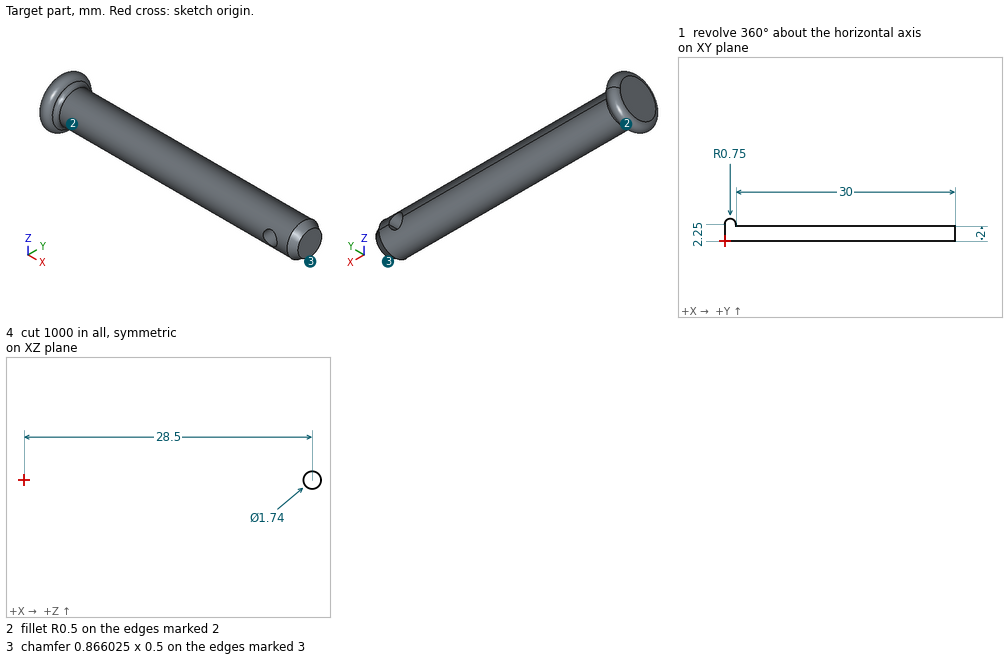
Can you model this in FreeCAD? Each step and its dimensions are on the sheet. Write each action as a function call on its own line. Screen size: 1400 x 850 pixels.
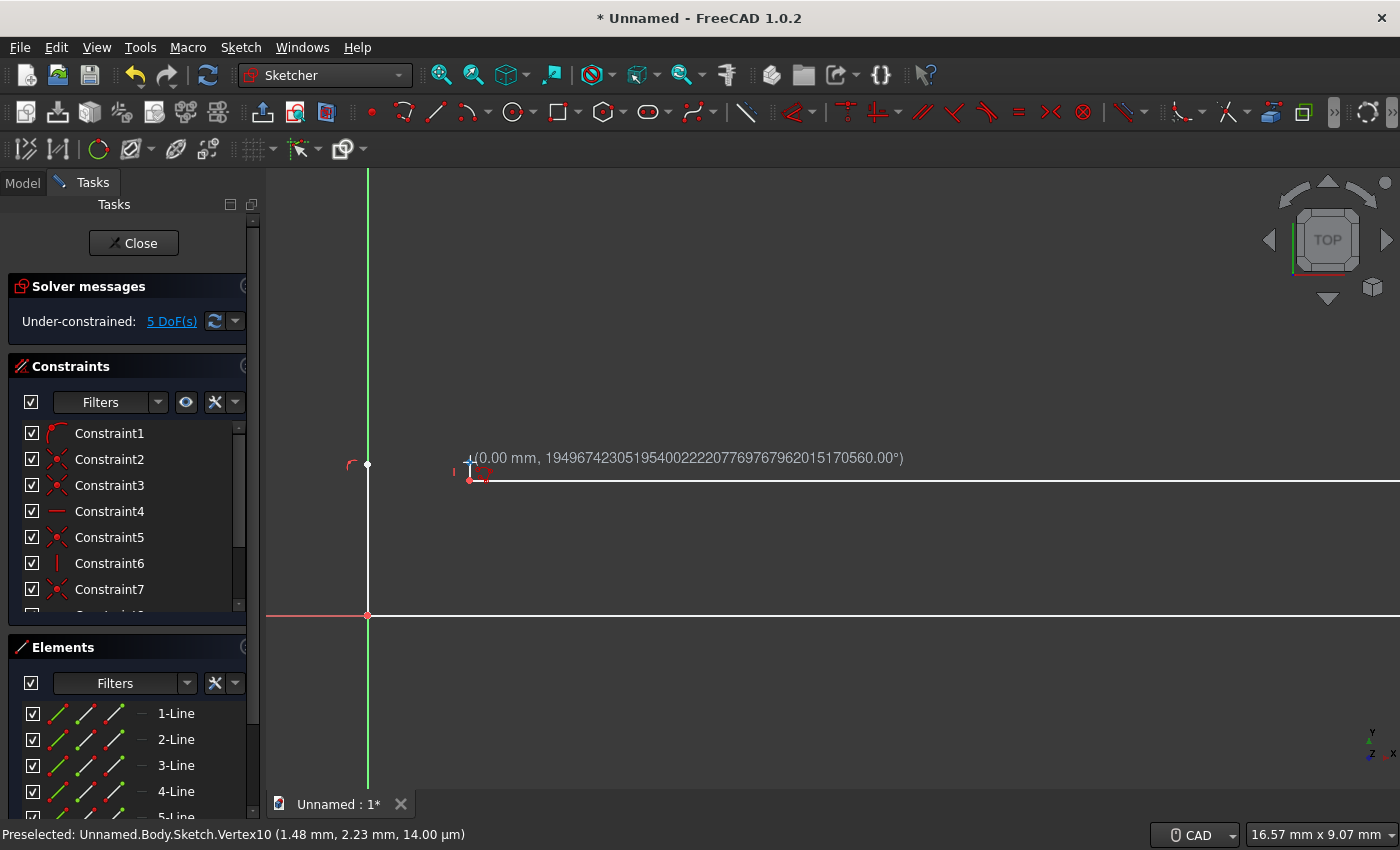
key(g)
key(3)
key(a)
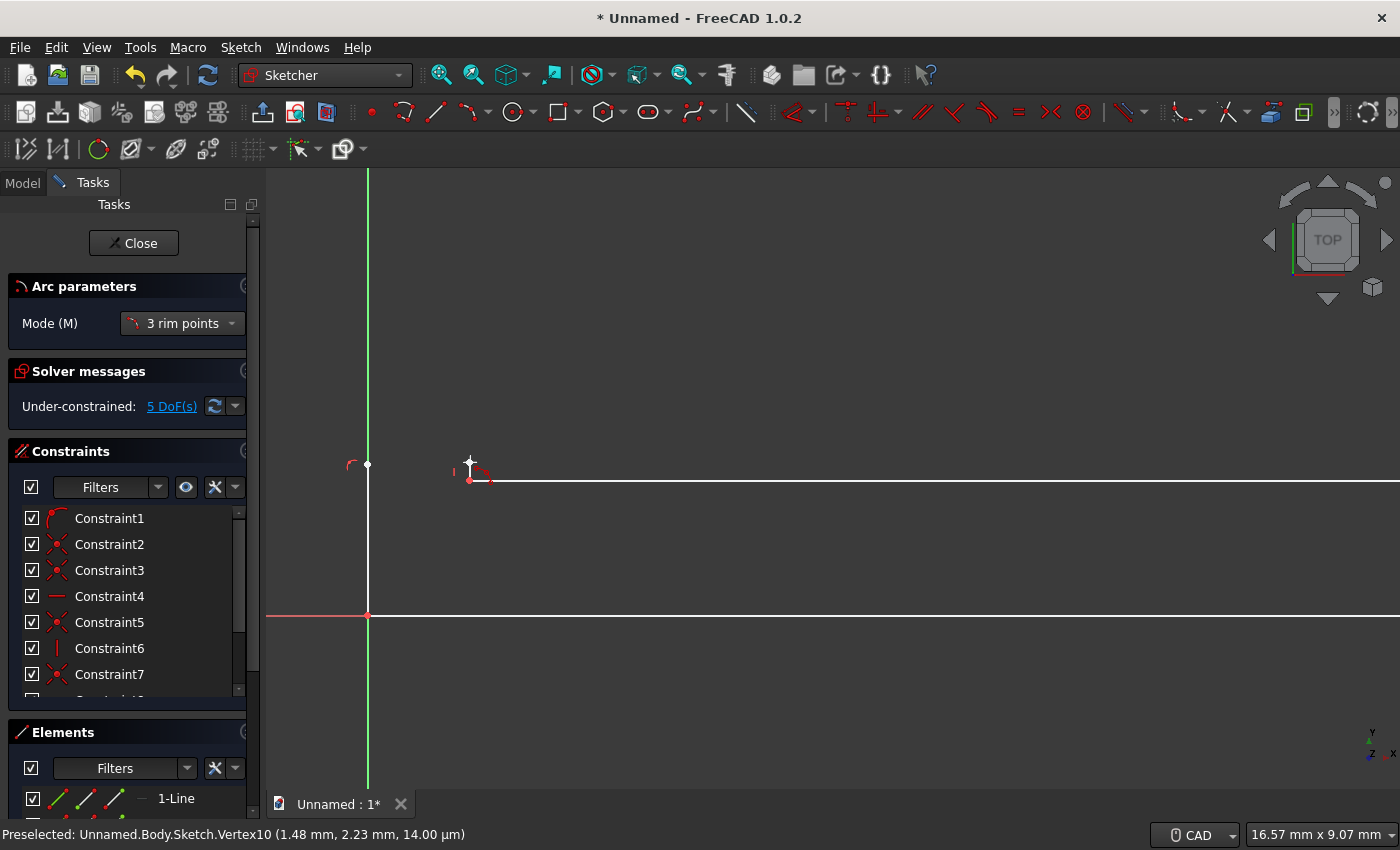
scroll(471, 462, up, 4)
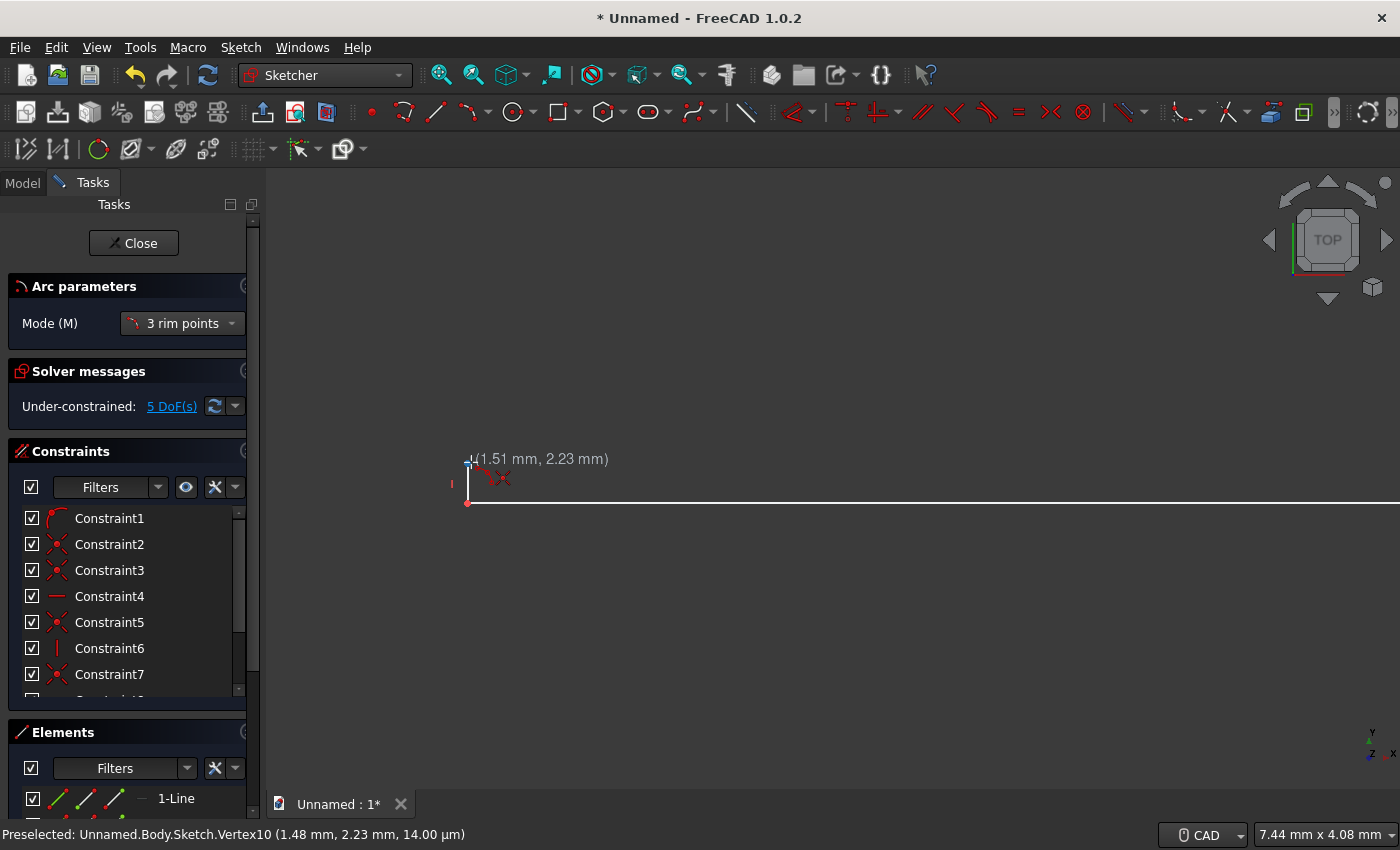
click(468, 464)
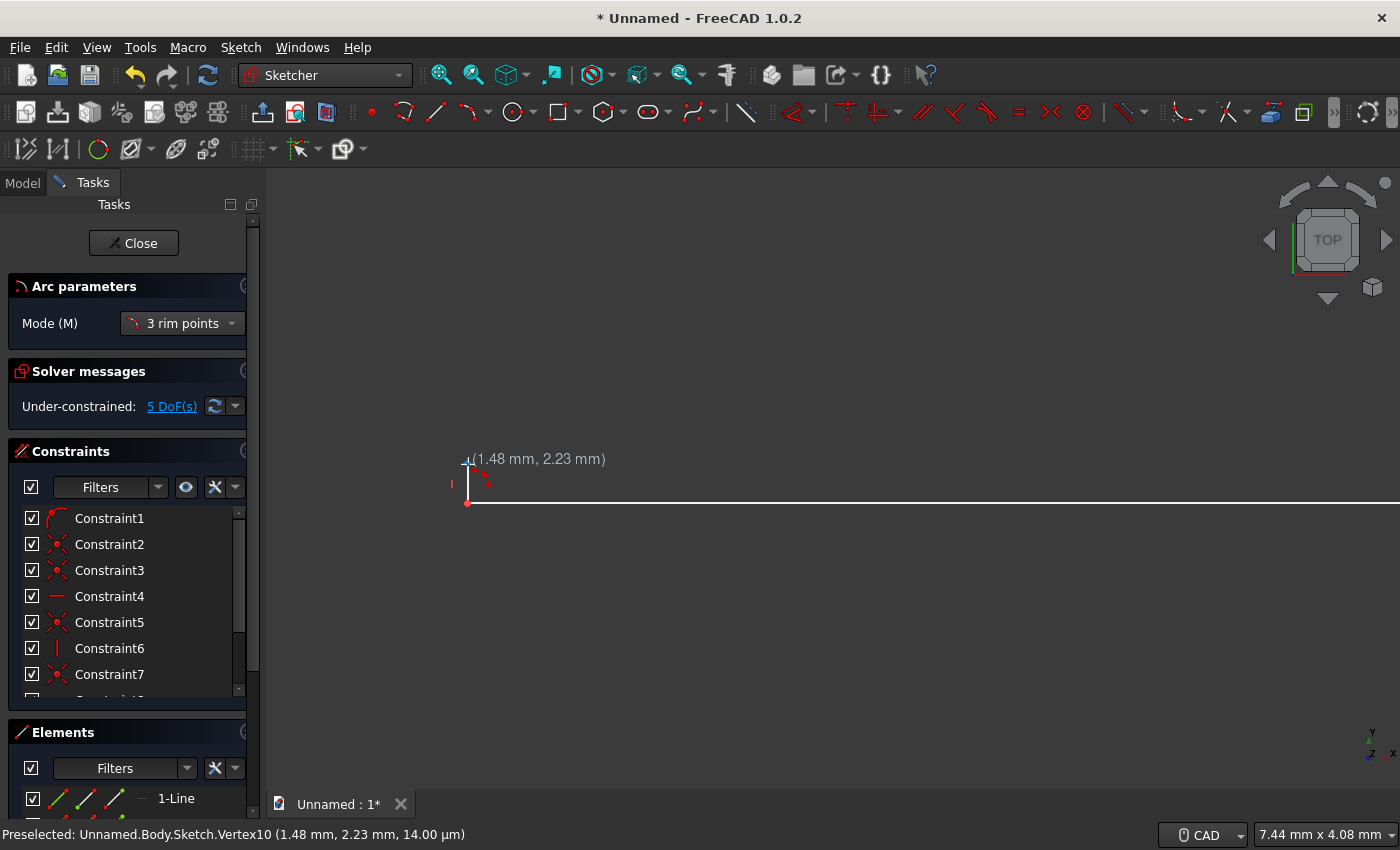
scroll(471, 463, down, 10)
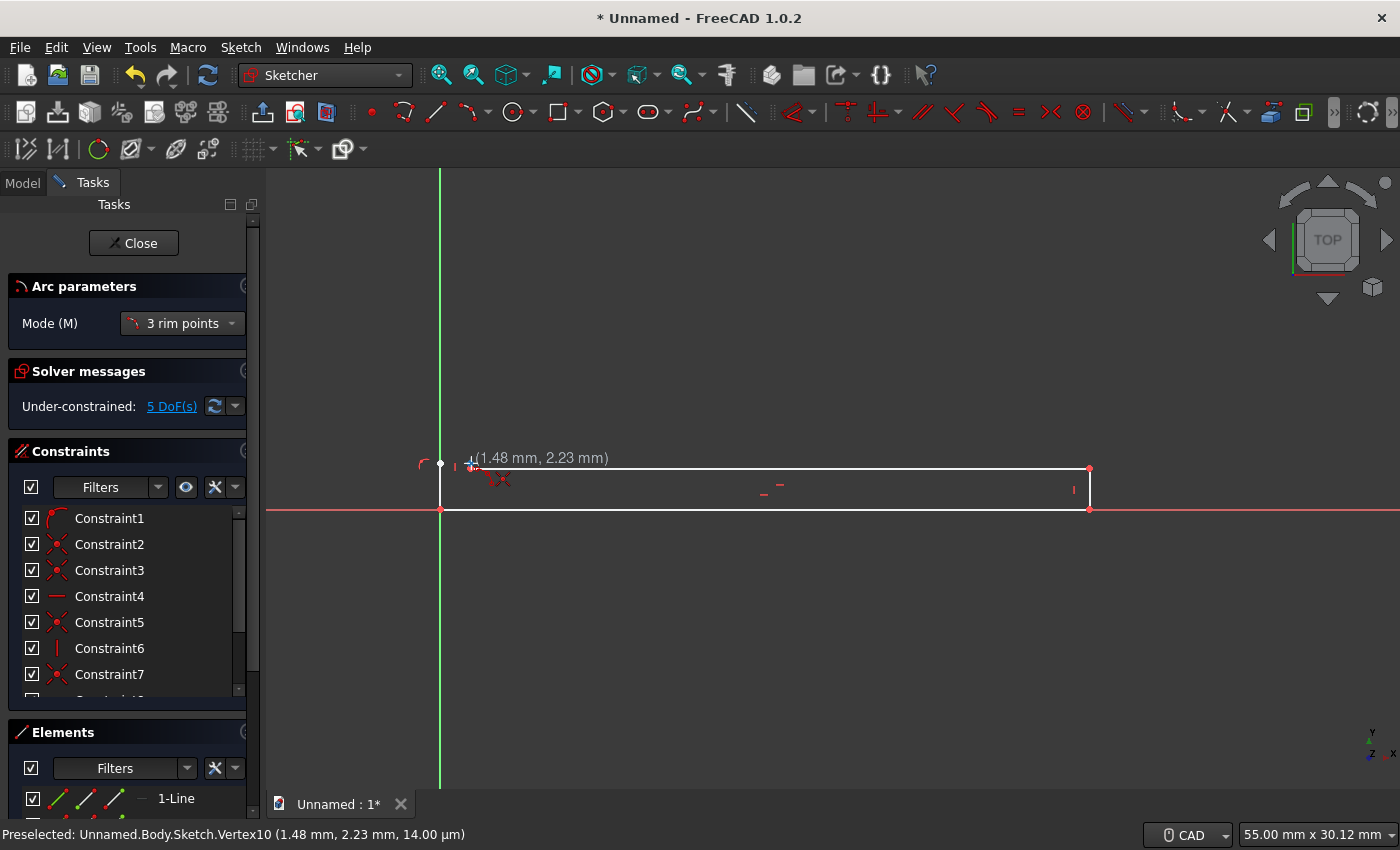
click(440, 464)
click(456, 448)
key(Escape)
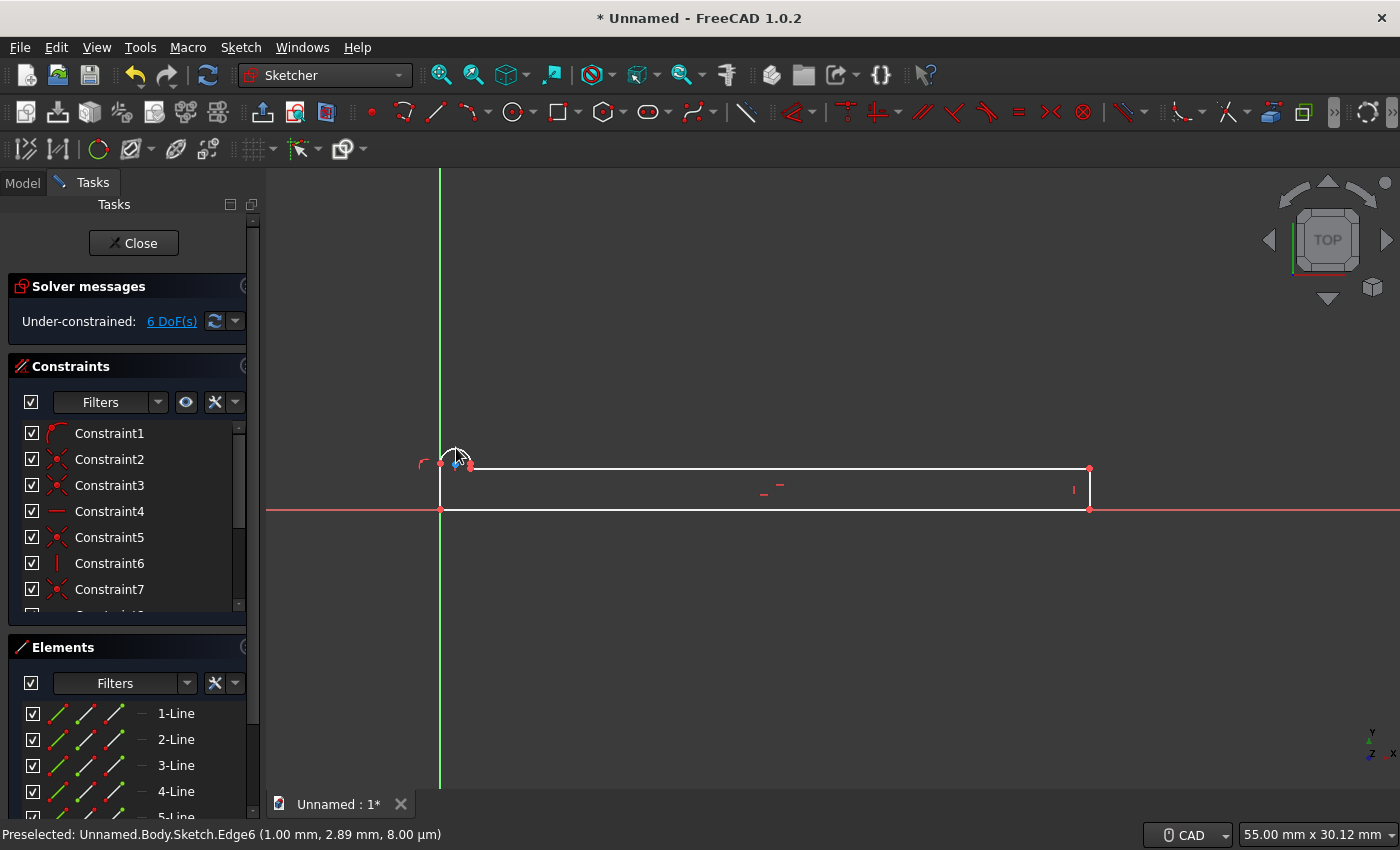
click(440, 478)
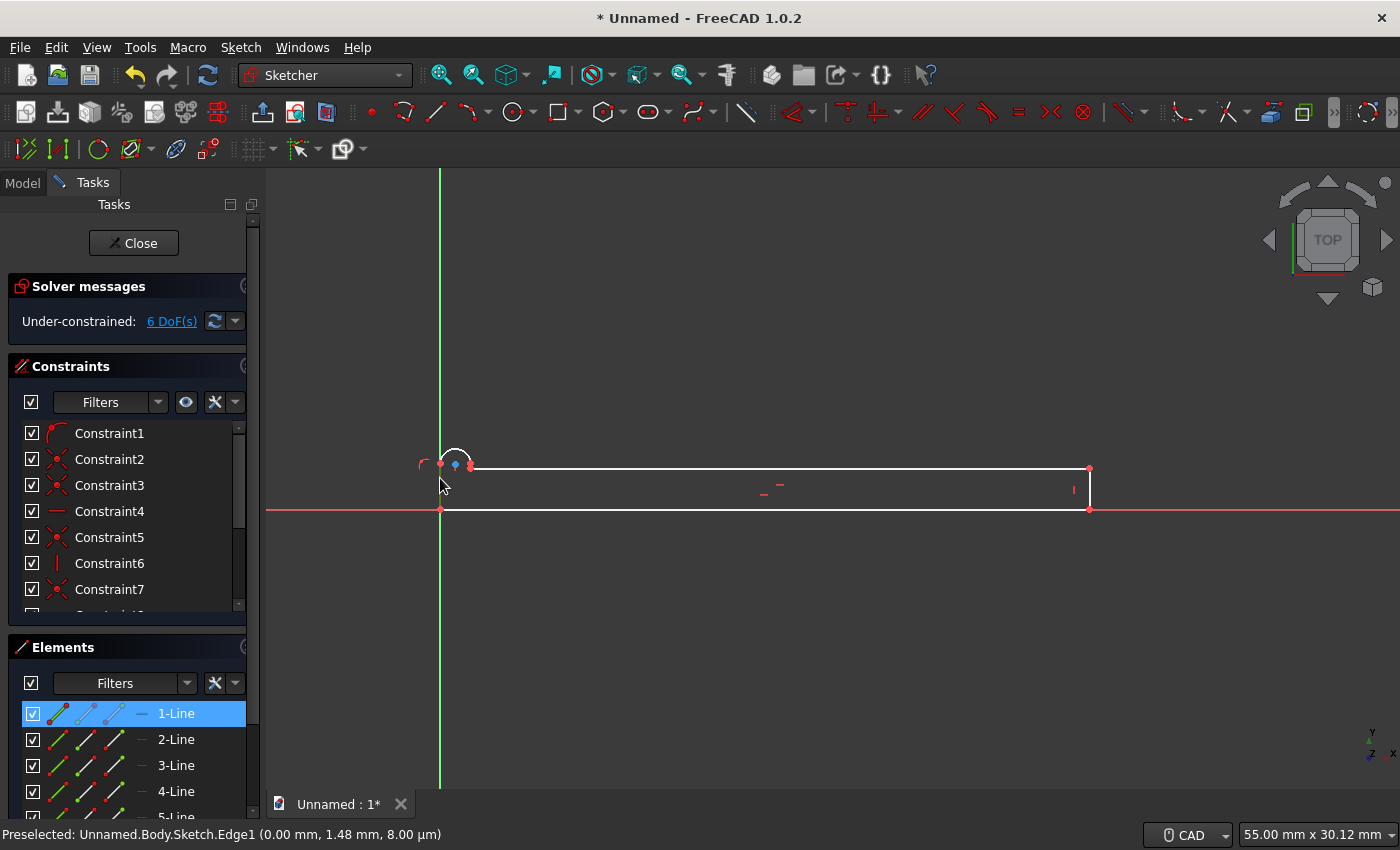
click(464, 452)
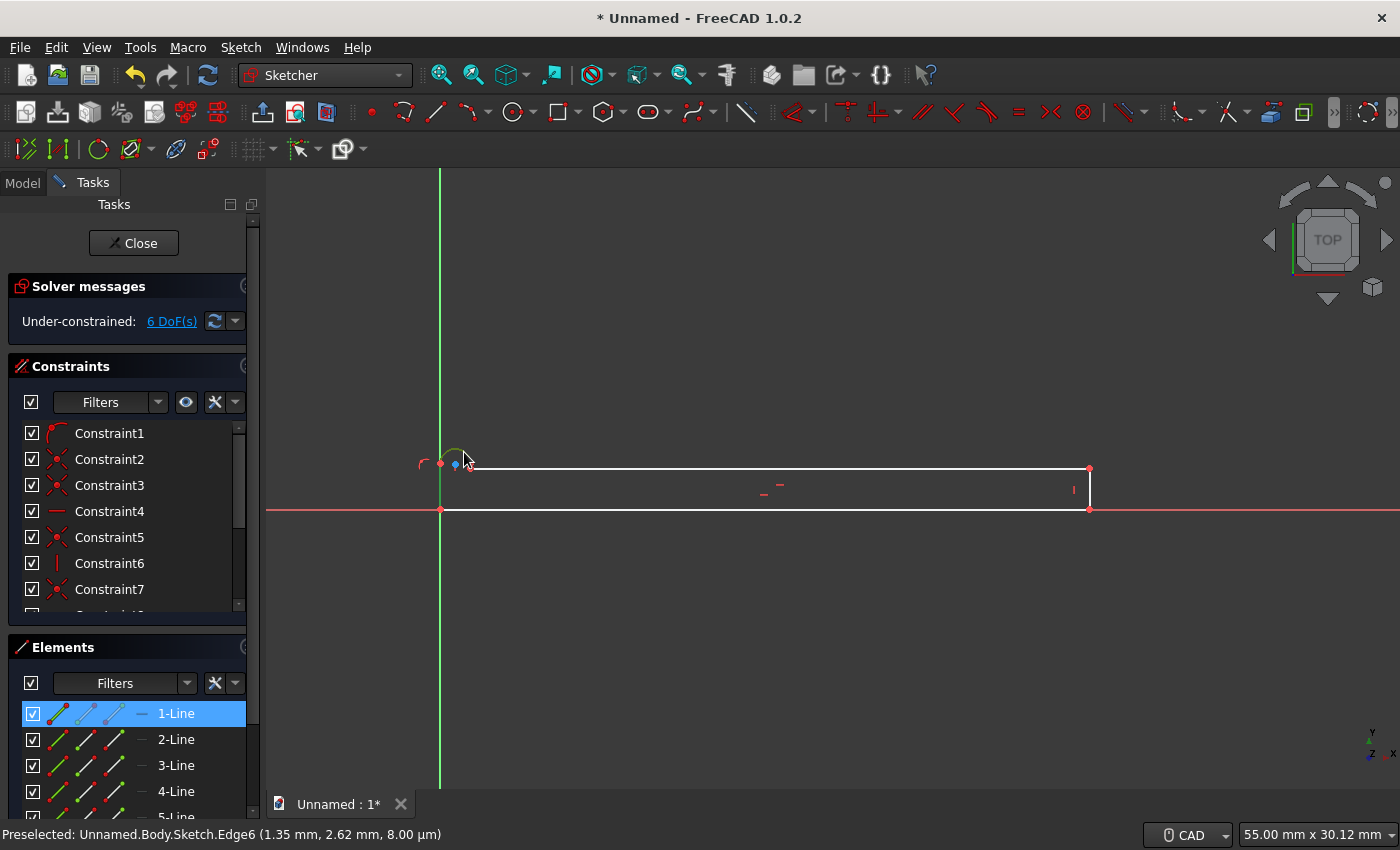
click(988, 112)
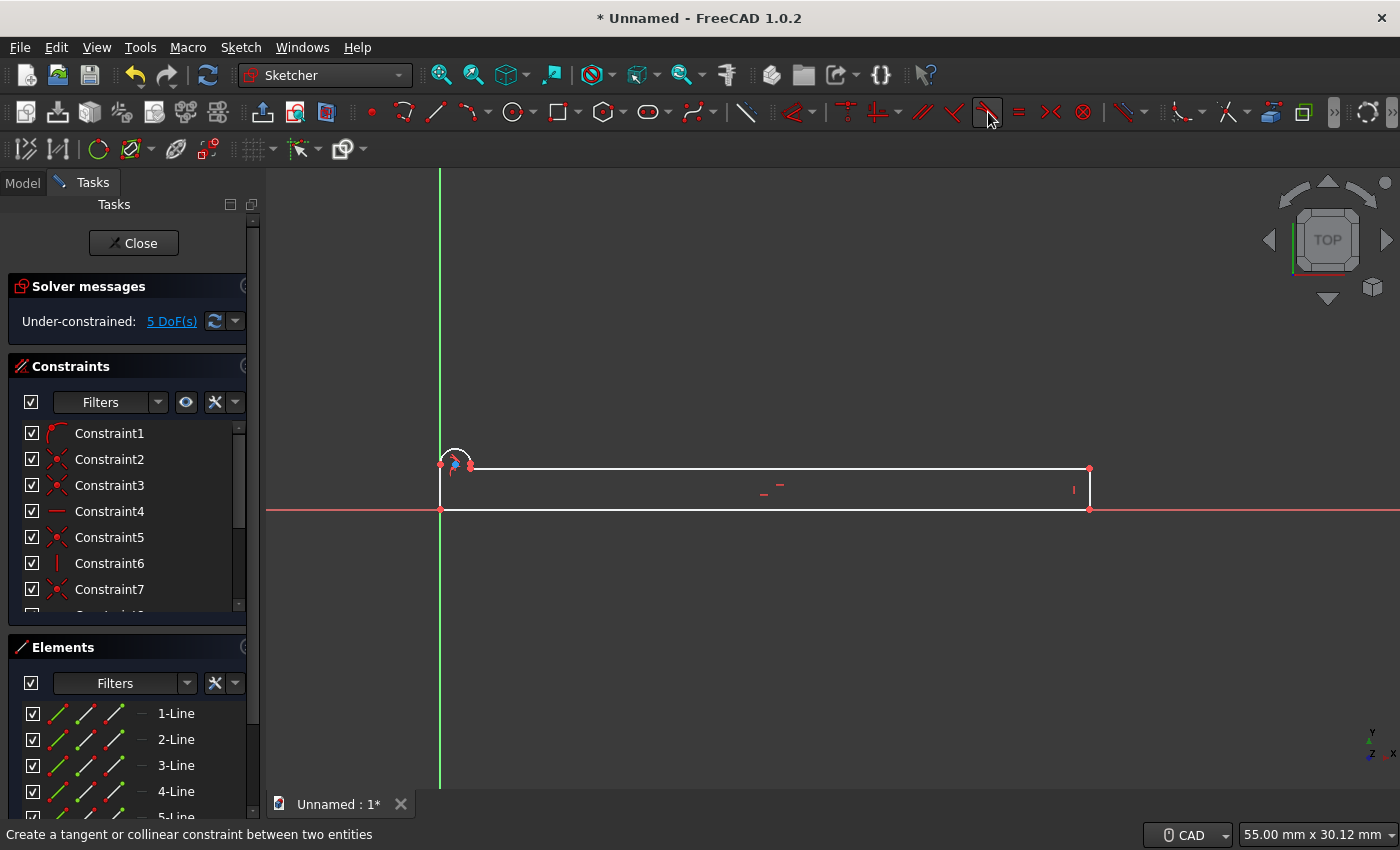
scroll(471, 466, up, 9)